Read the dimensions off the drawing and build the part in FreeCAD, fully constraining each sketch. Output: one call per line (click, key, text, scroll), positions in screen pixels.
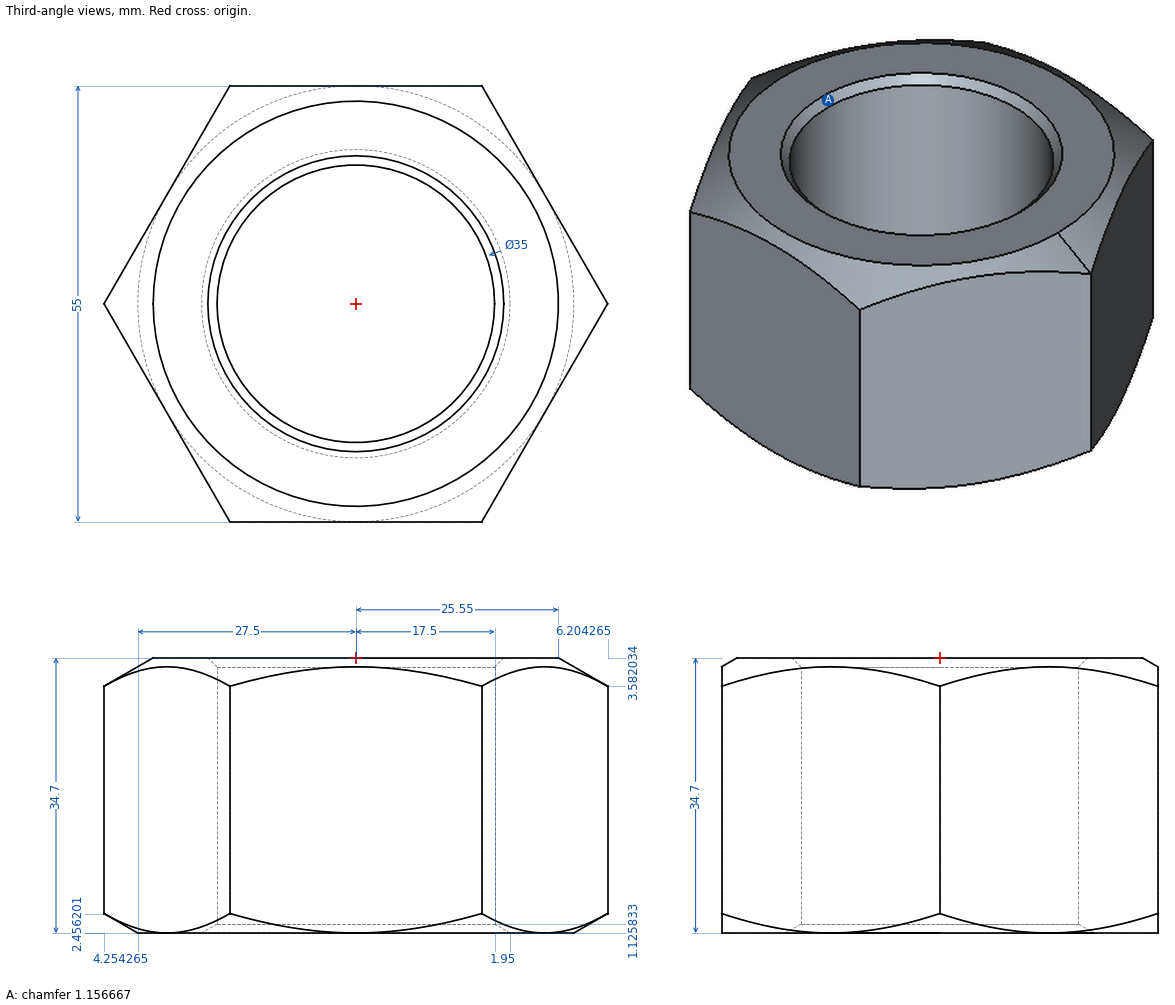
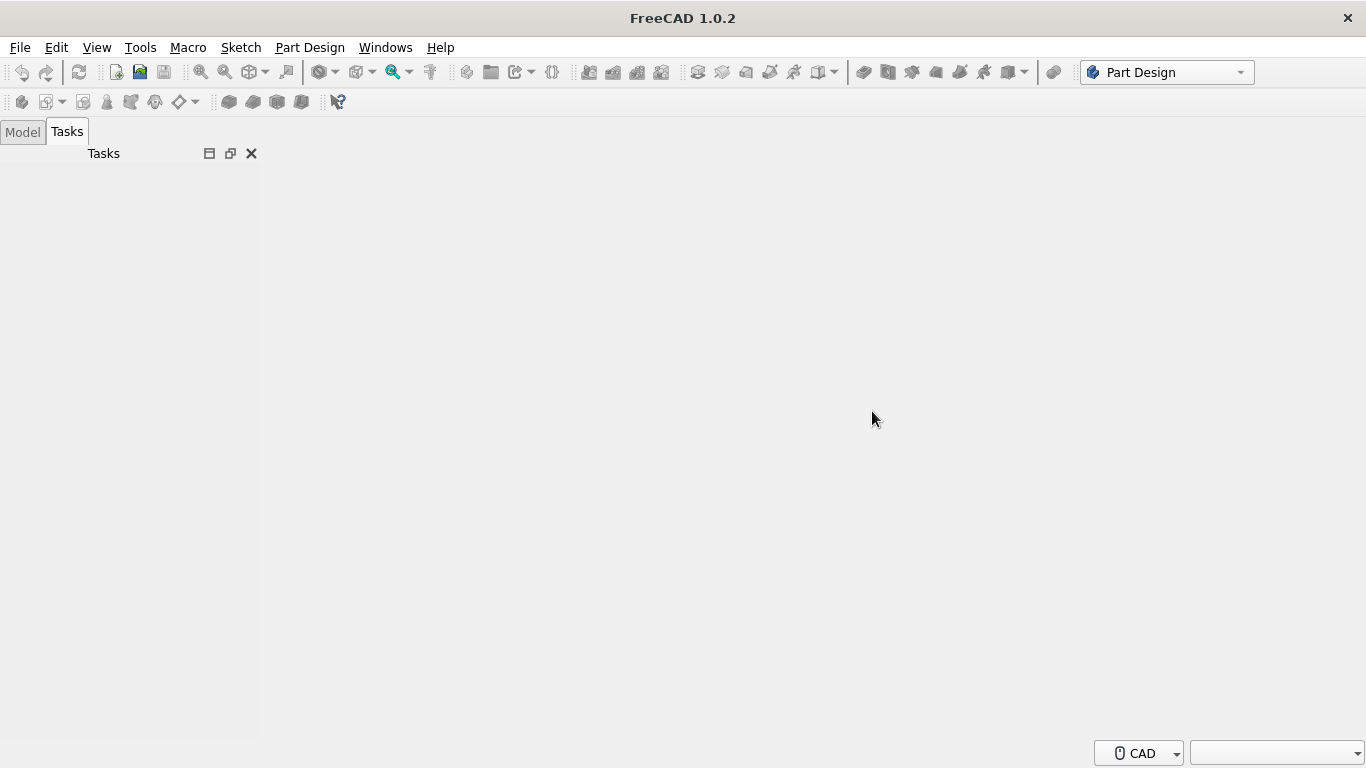
click(116, 72)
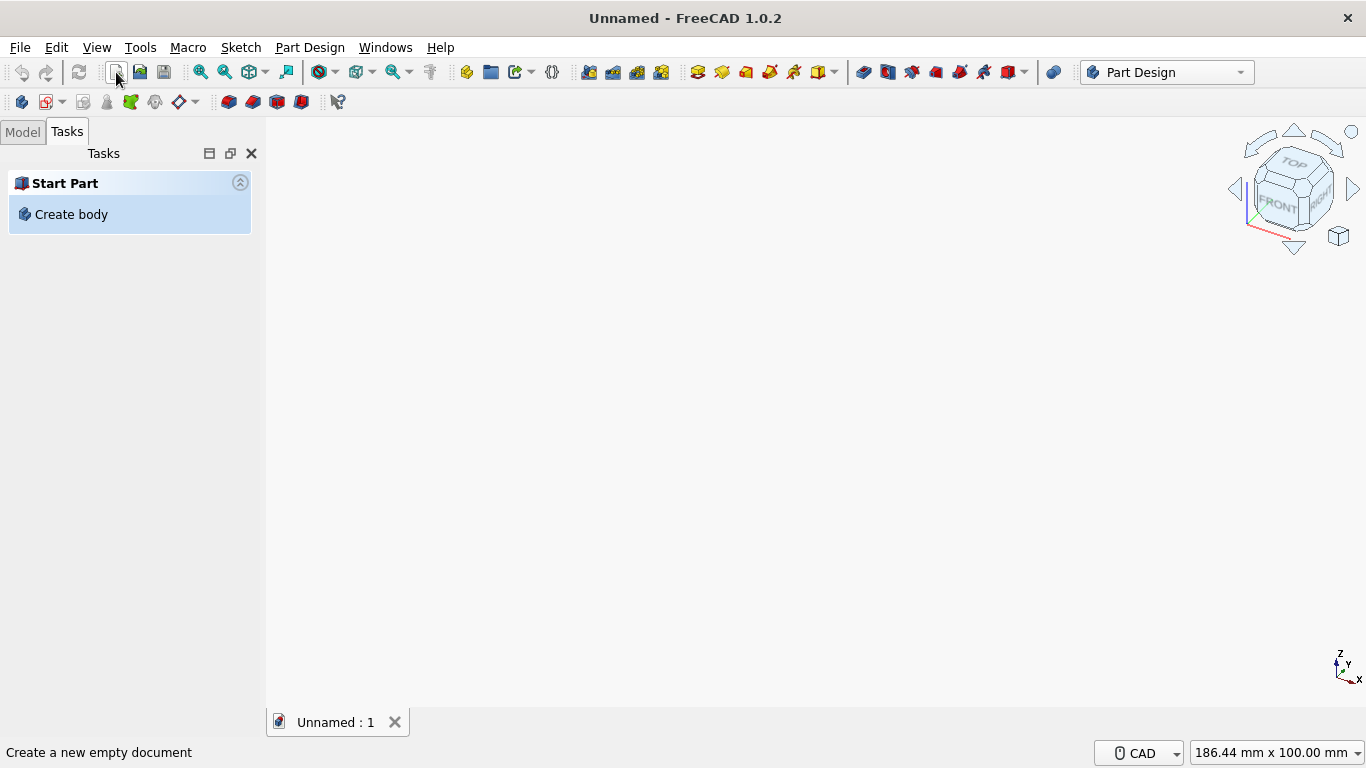
click(46, 102)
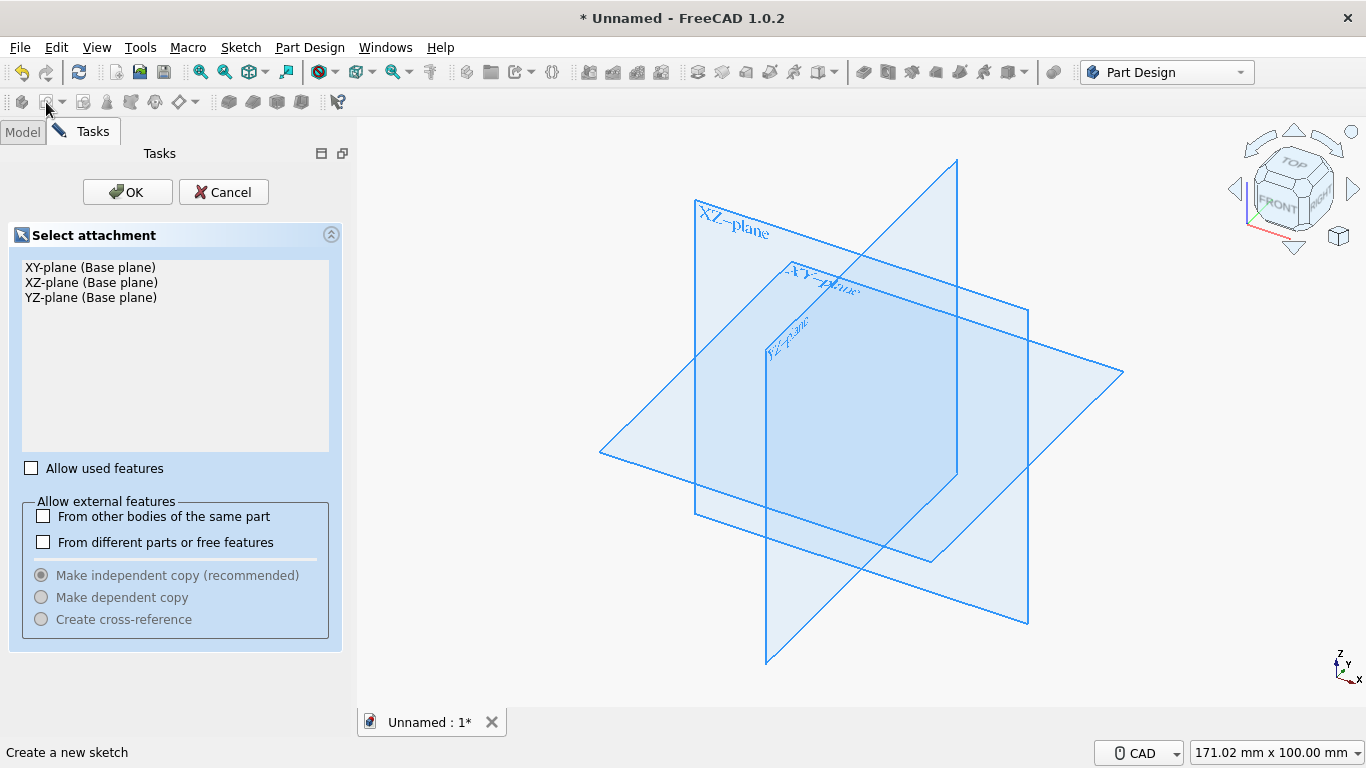
click(82, 268)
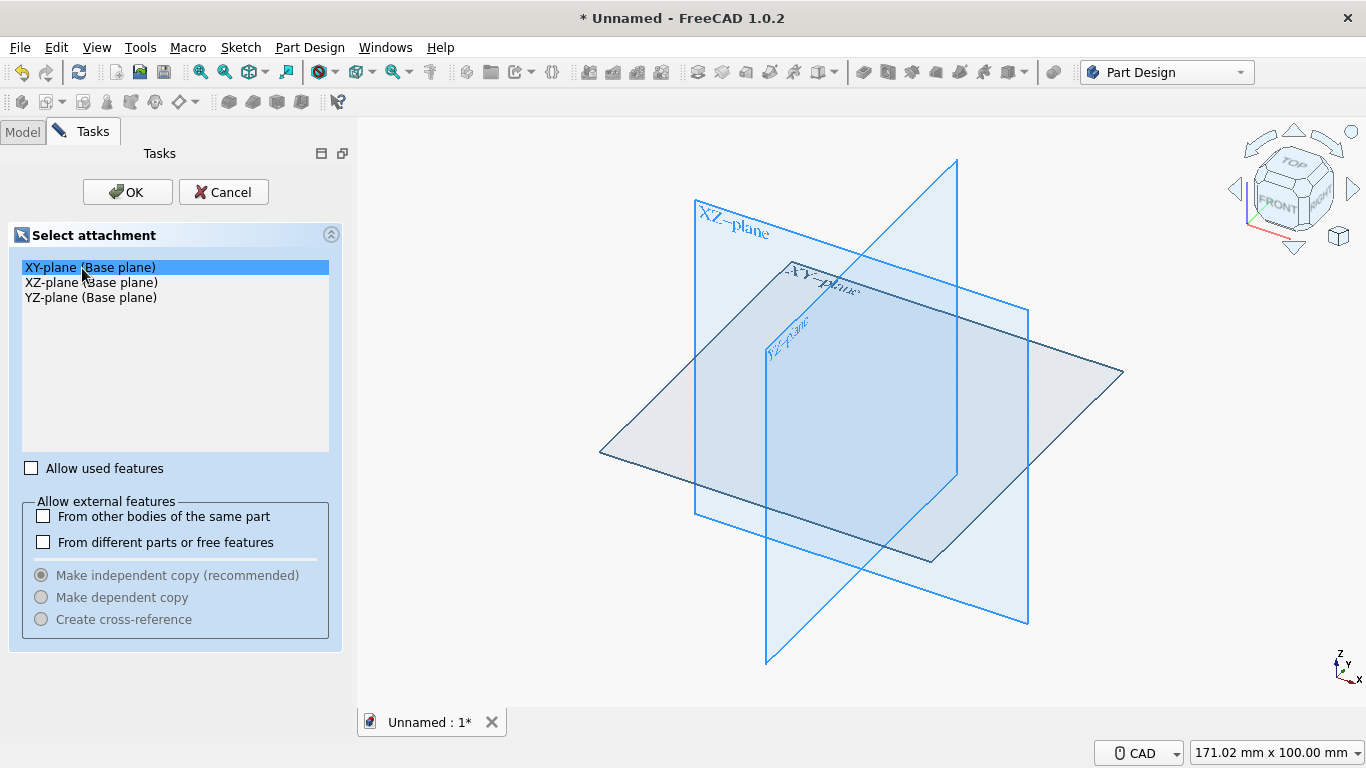
click(128, 192)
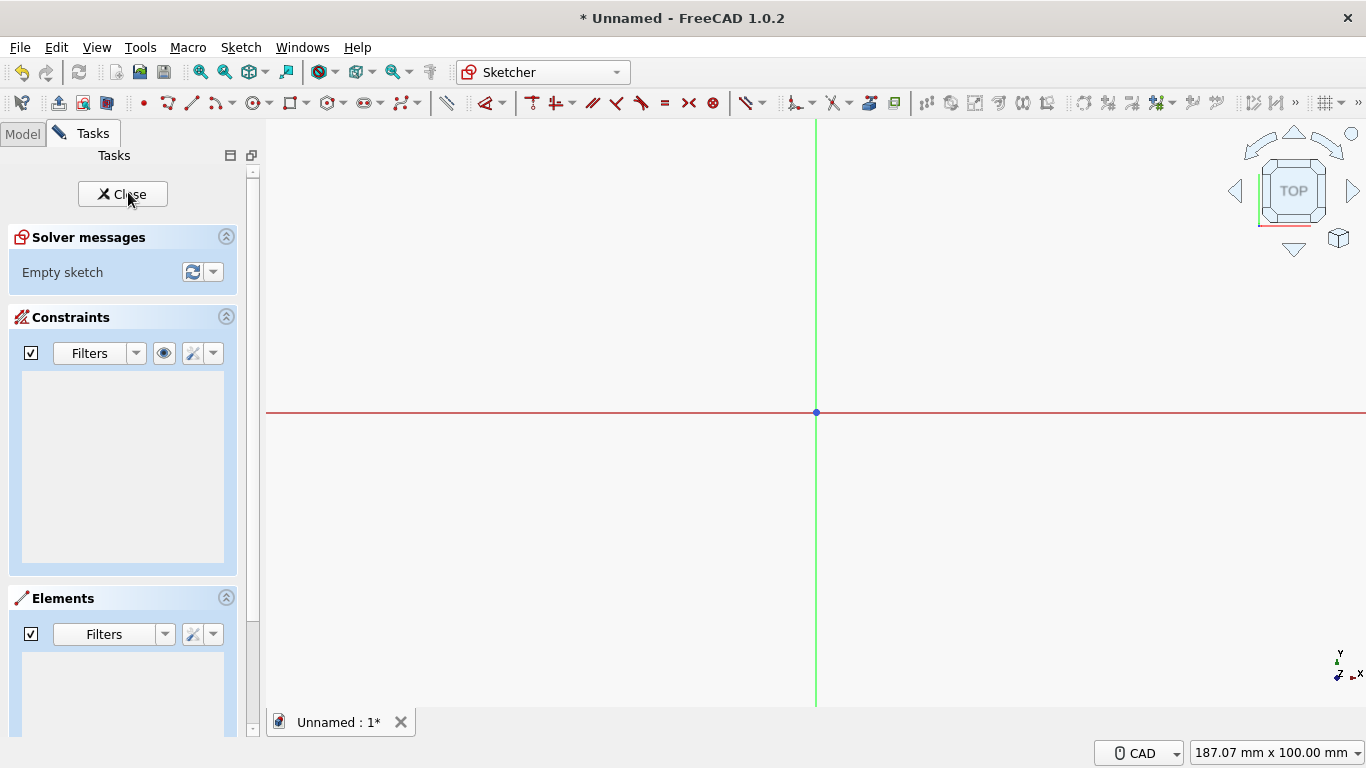
key(g)
key(p)
key(6)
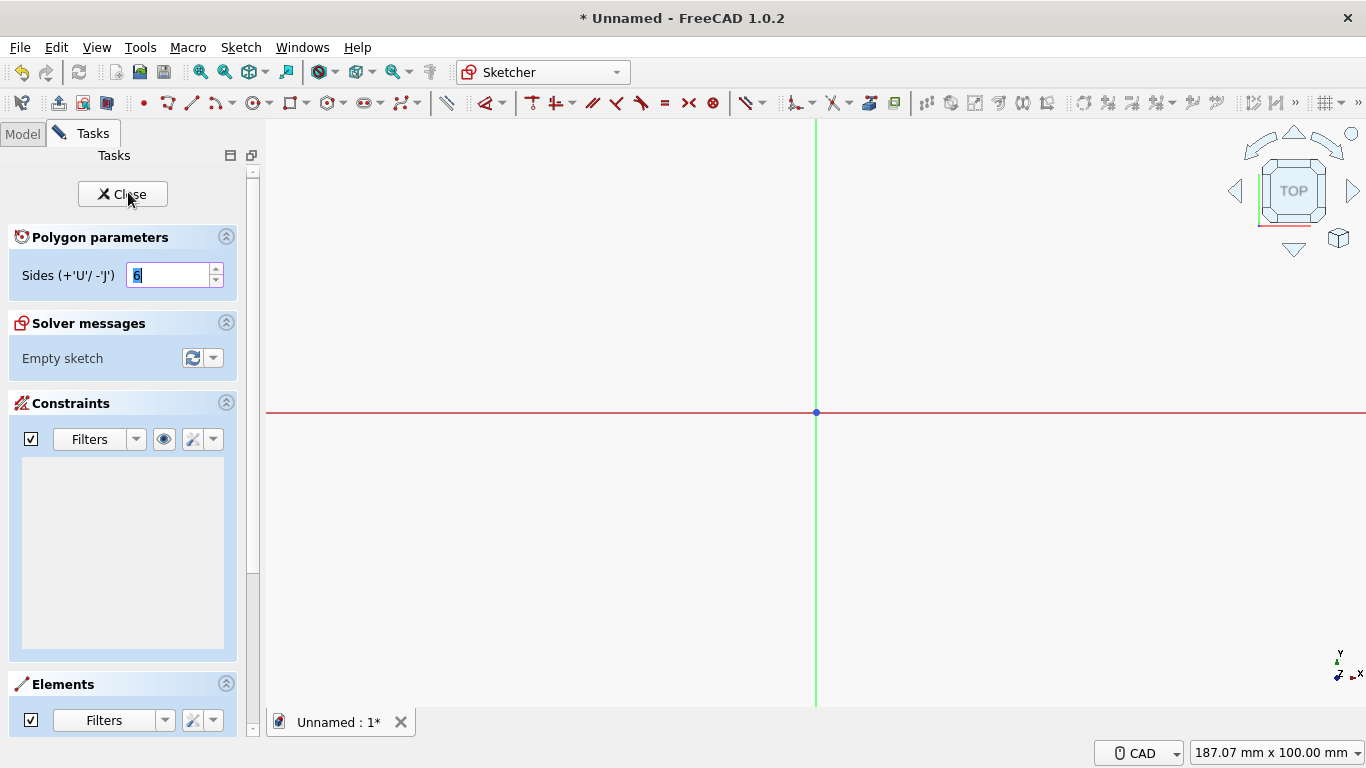
click(816, 413)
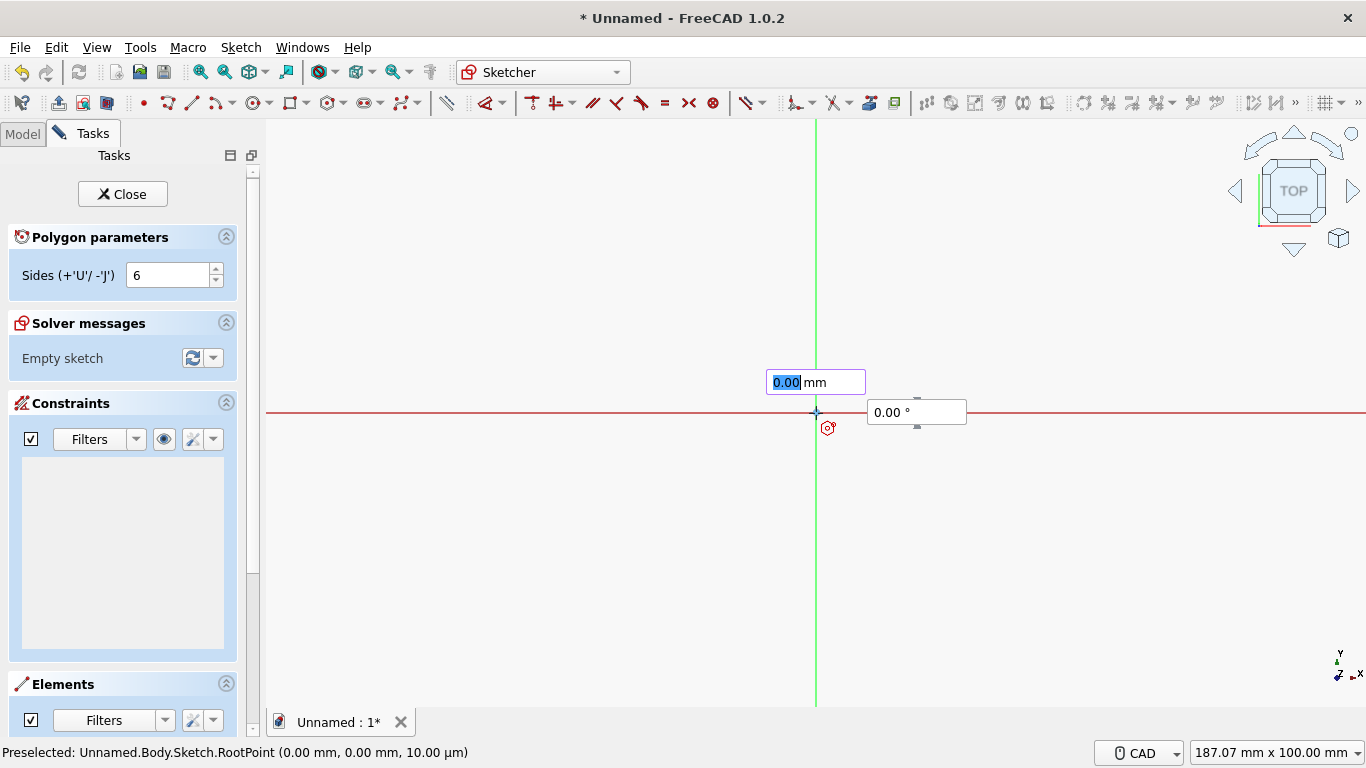
click(1003, 413)
right_click(1003, 413)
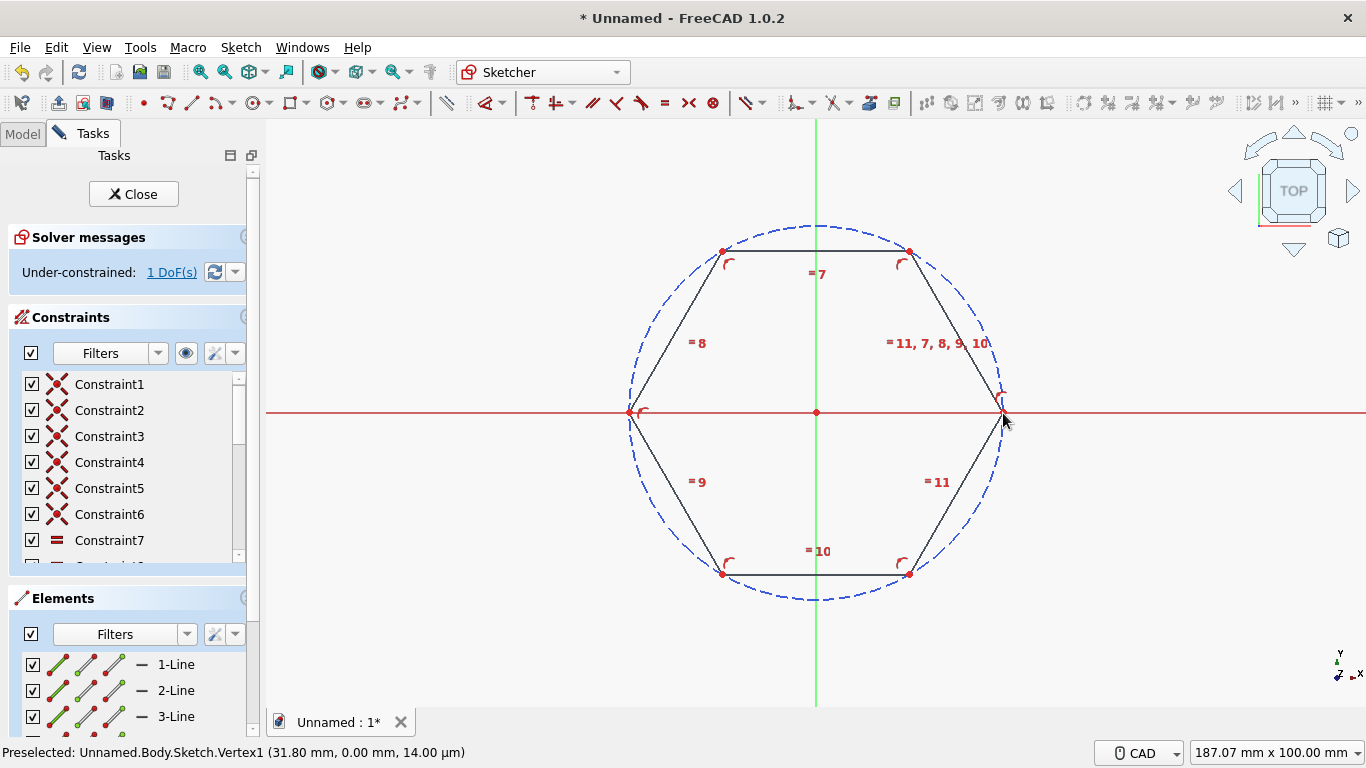
click(254, 104)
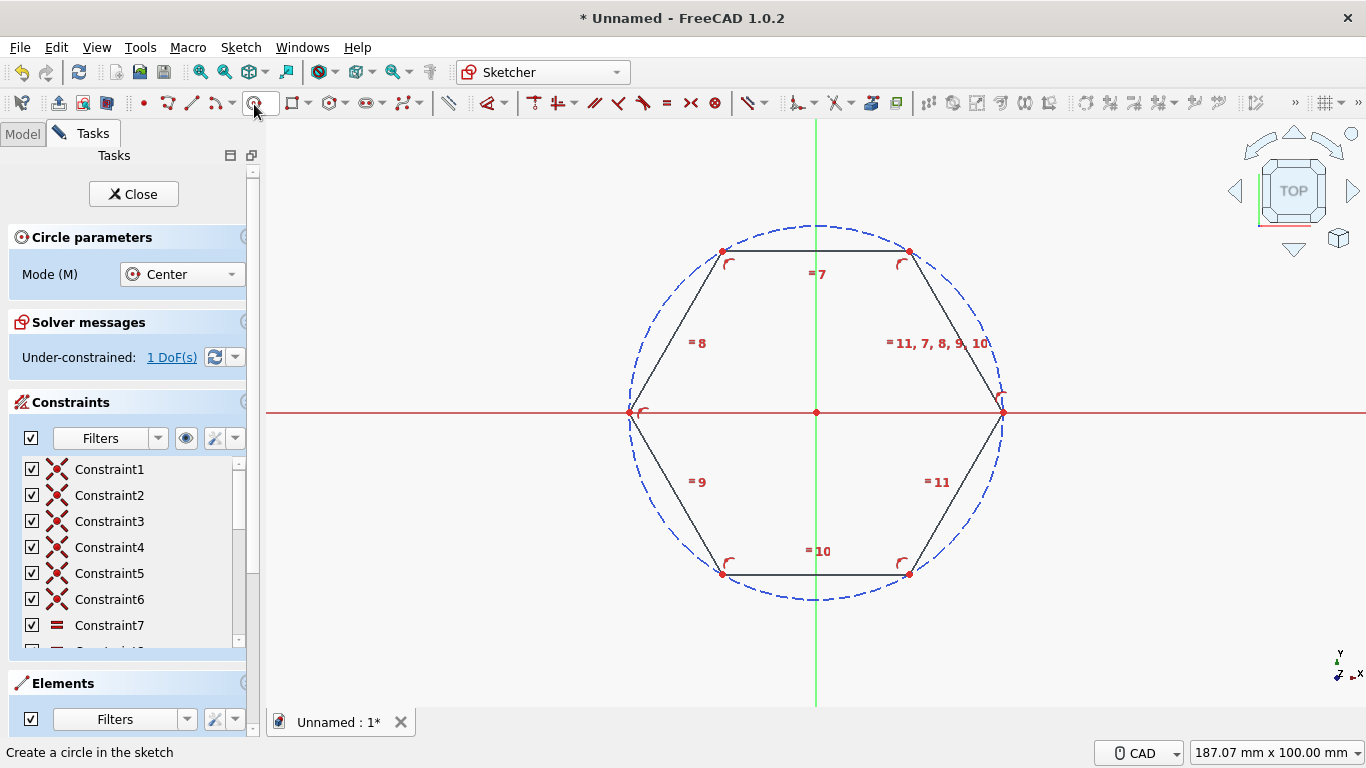
click(816, 413)
move(889, 340)